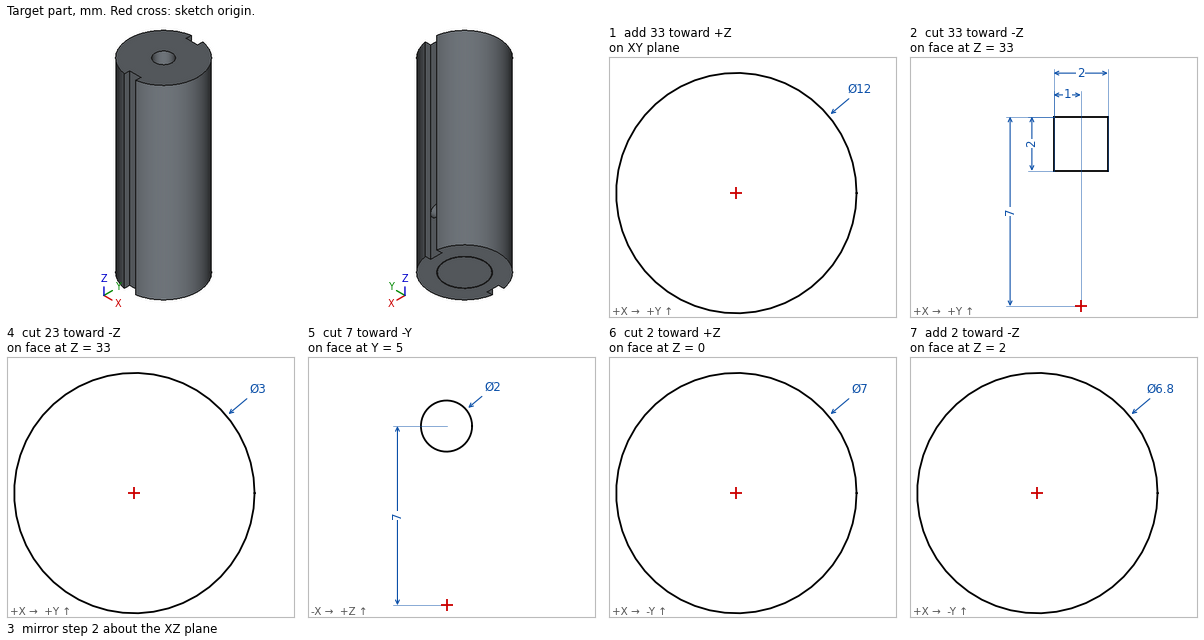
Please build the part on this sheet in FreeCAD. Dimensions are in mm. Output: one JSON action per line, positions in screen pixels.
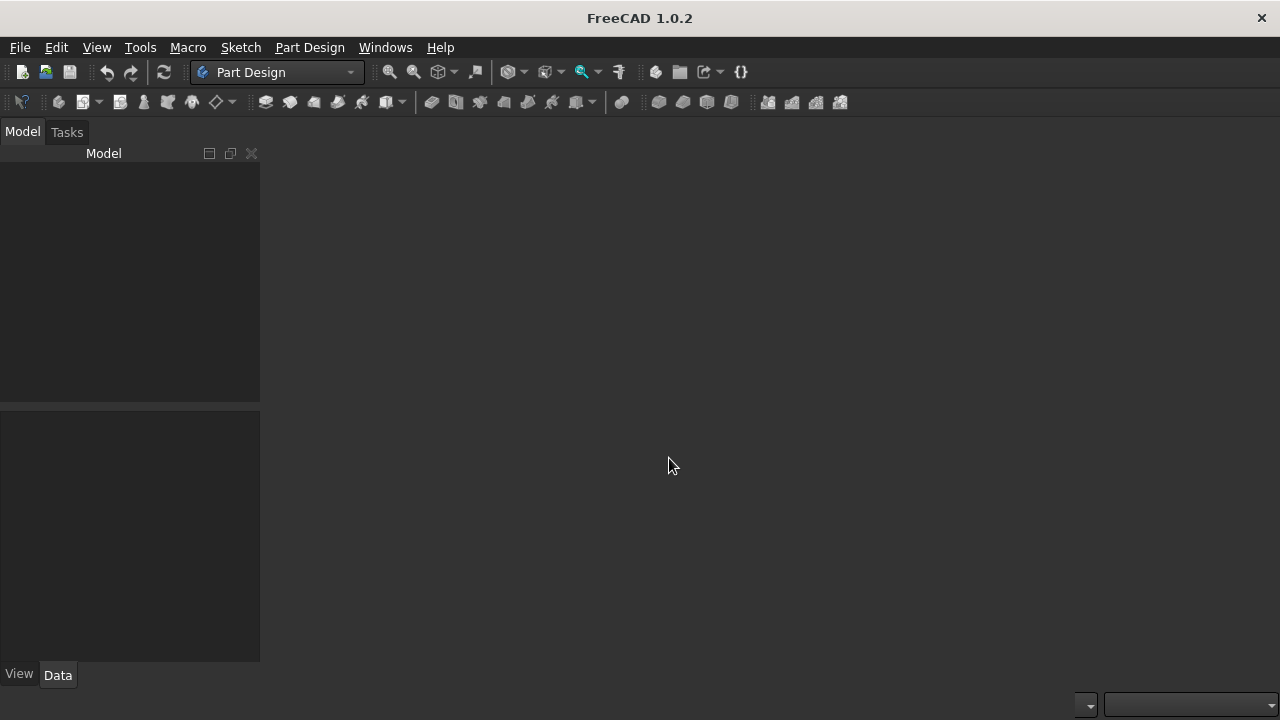
{"action": "key", "text": "ctrl+n"}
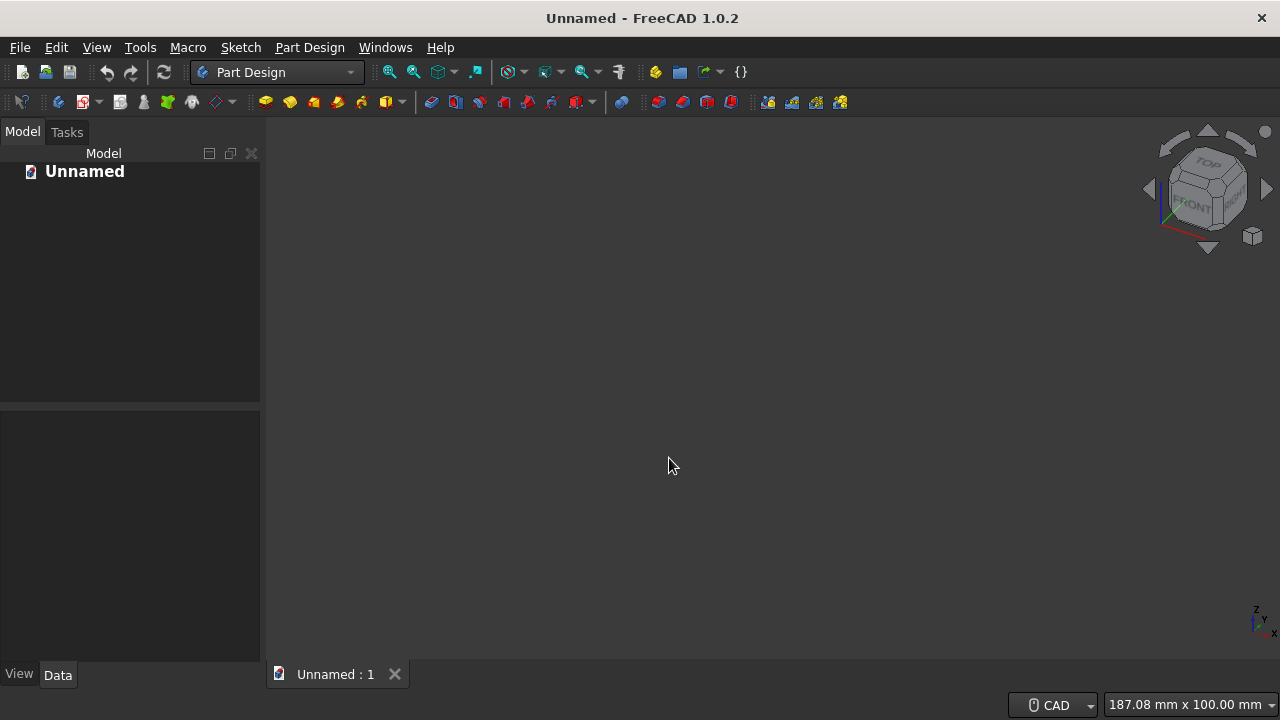
{"action": "left_click", "coordinate": [84, 102]}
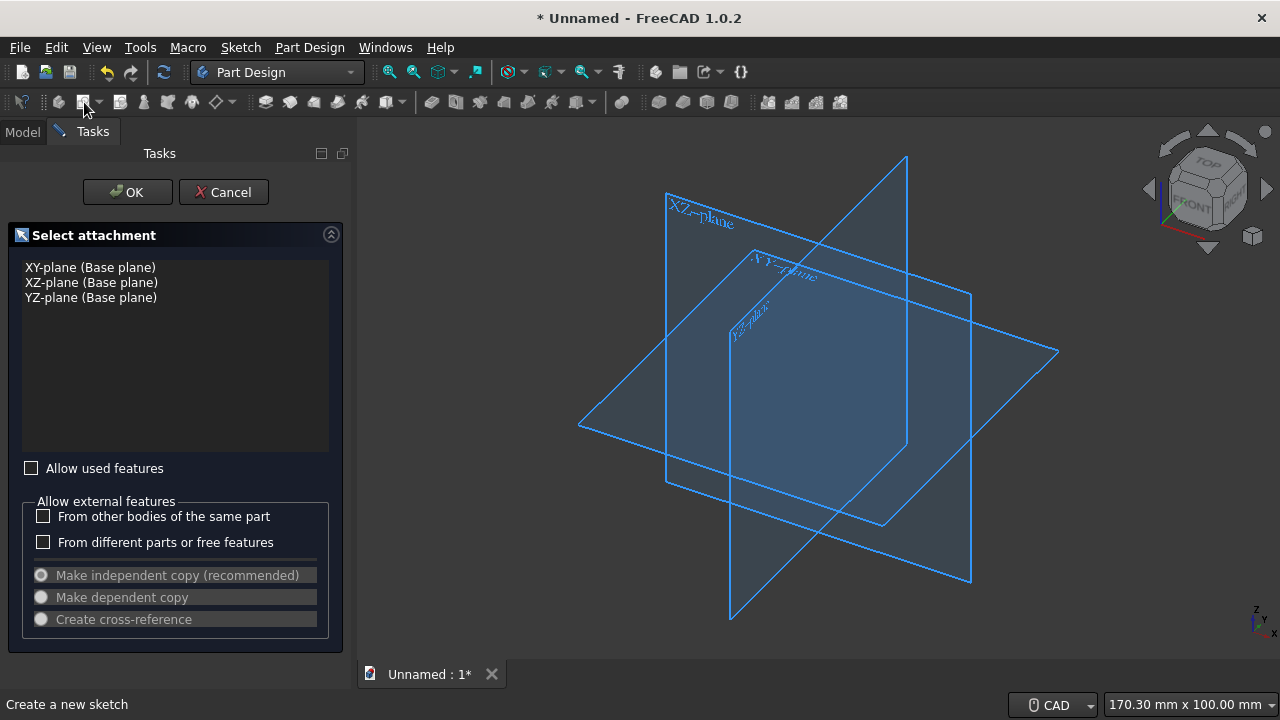
{"action": "left_click", "coordinate": [82, 268]}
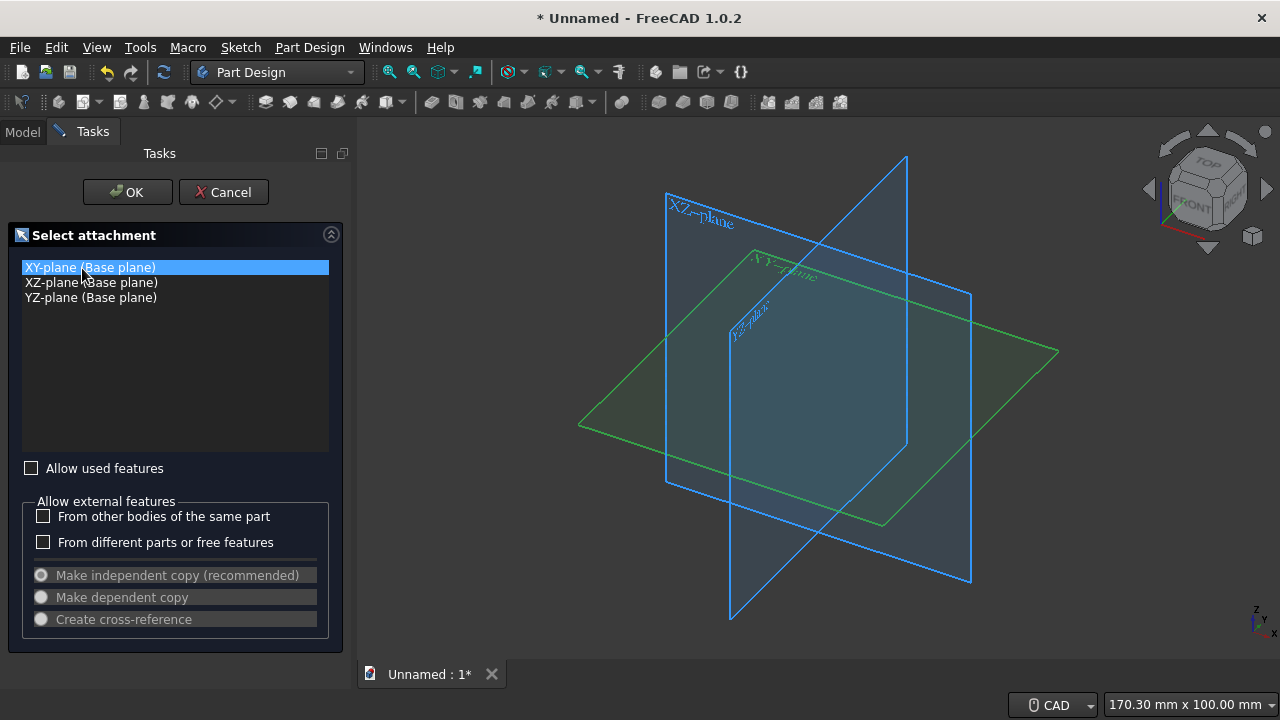
{"action": "left_click", "coordinate": [128, 192]}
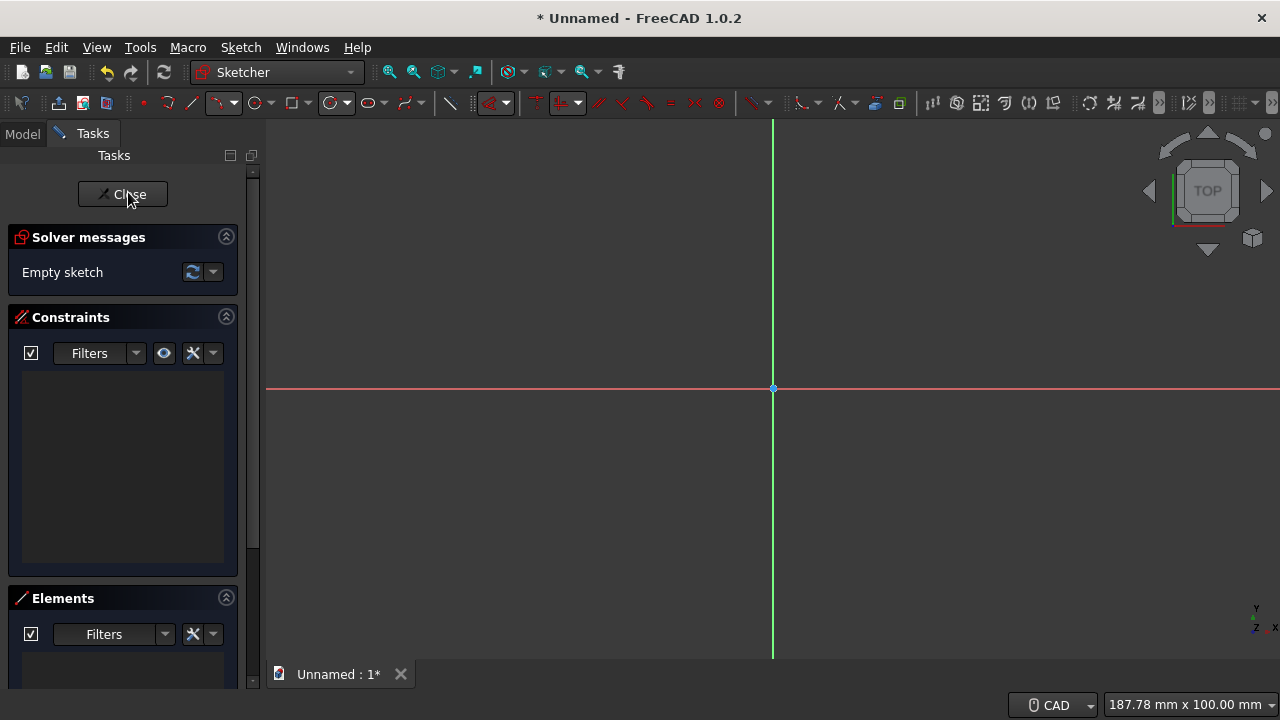
{"action": "scroll", "coordinate": [790, 389], "scroll_direction": "up", "scroll_amount": 8}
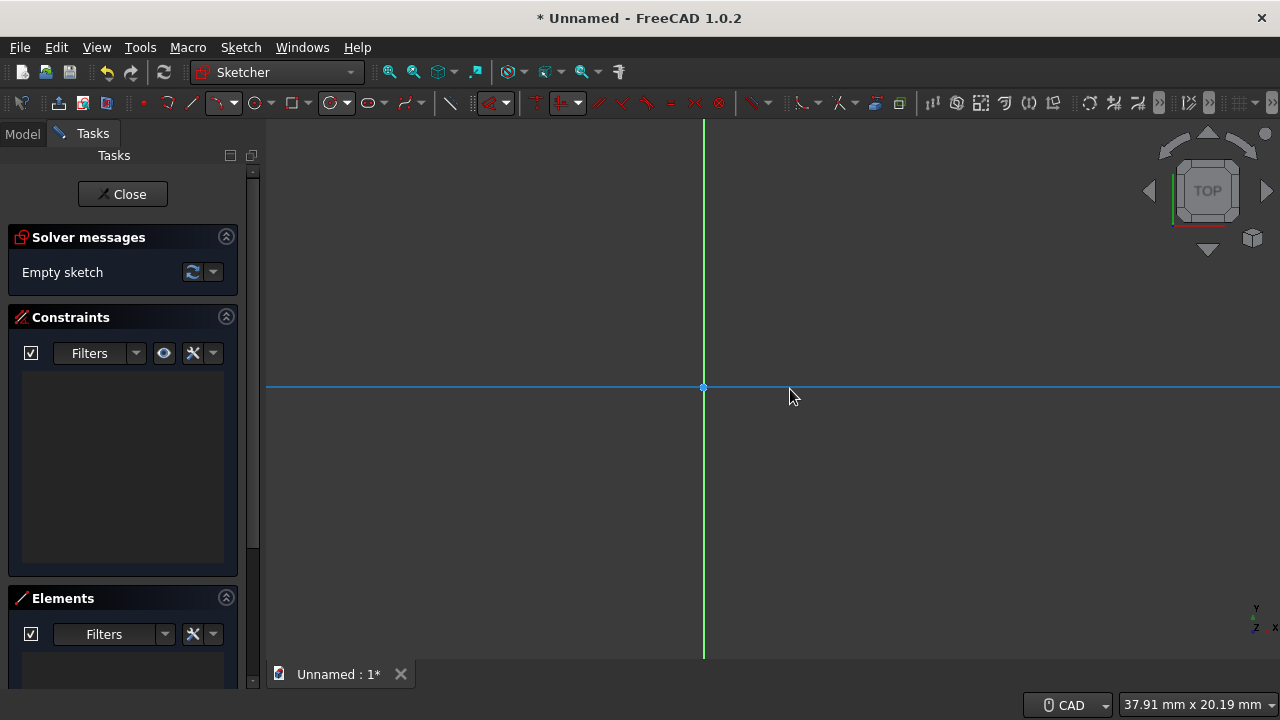
{"action": "key", "text": "g c"}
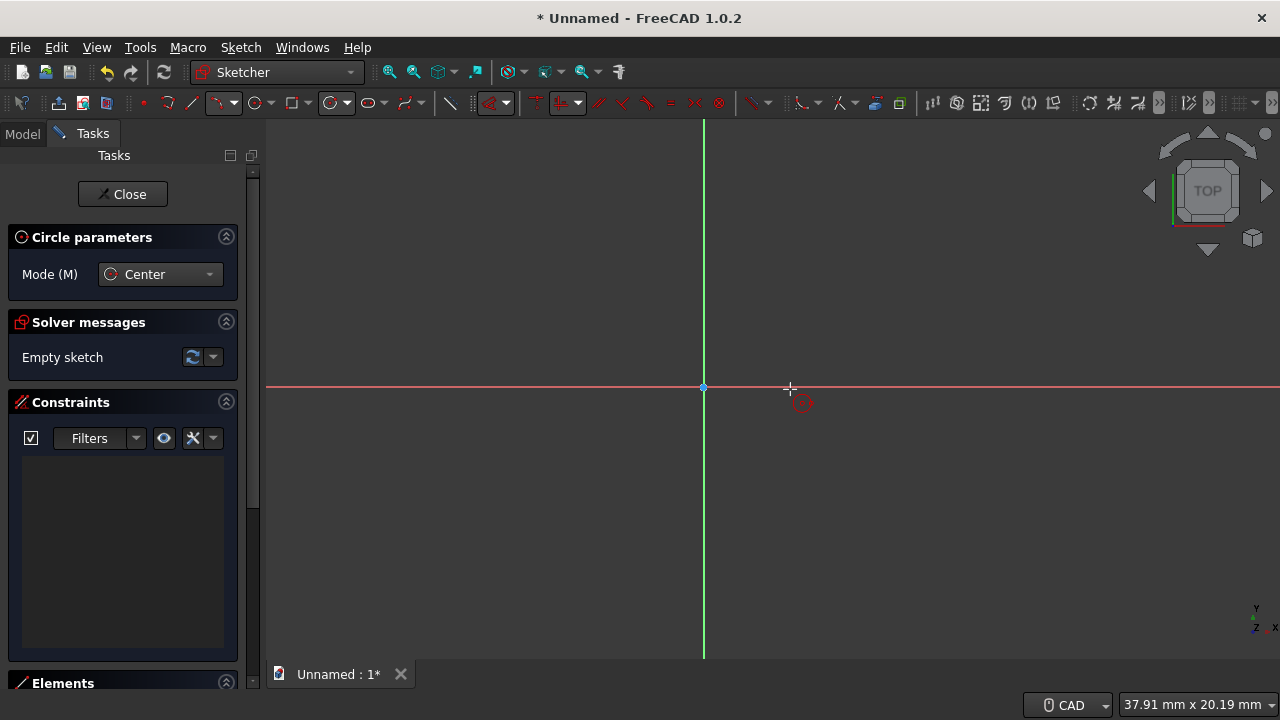
{"action": "left_click", "coordinate": [704, 387]}
{"action": "left_click", "coordinate": [817, 274]}
{"action": "key", "text": "Escape"}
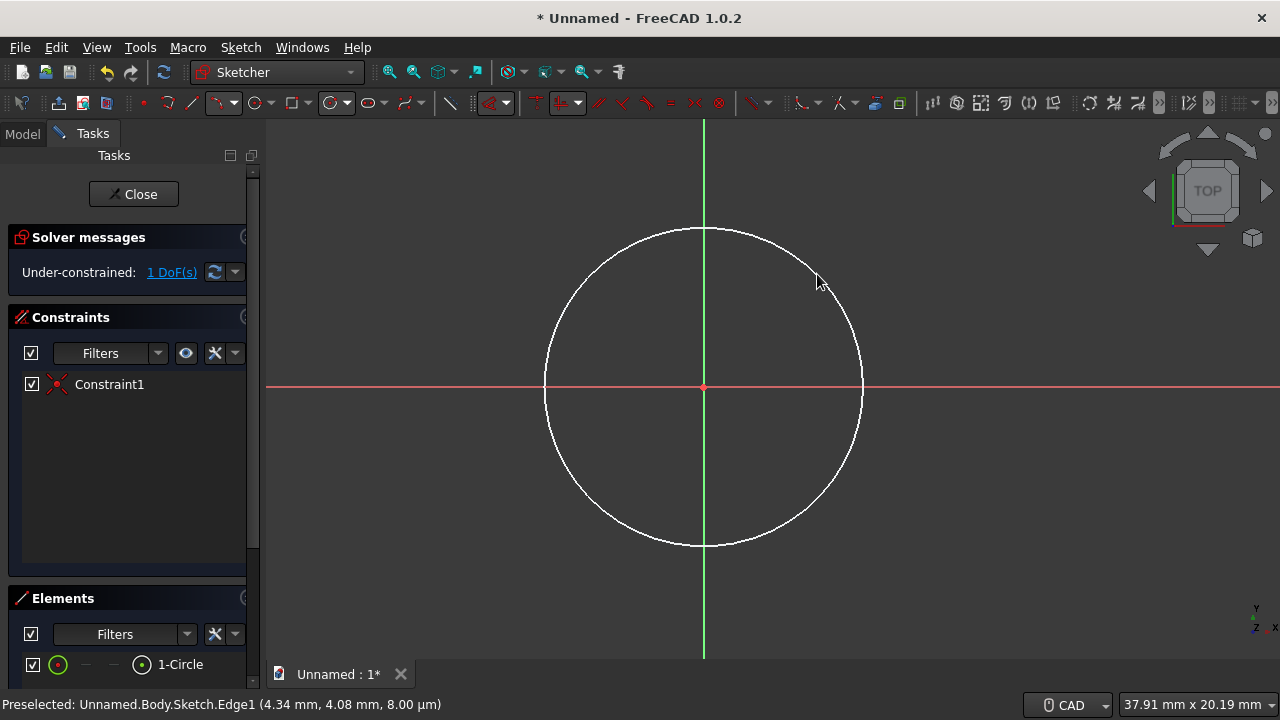
{"action": "key", "text": "d"}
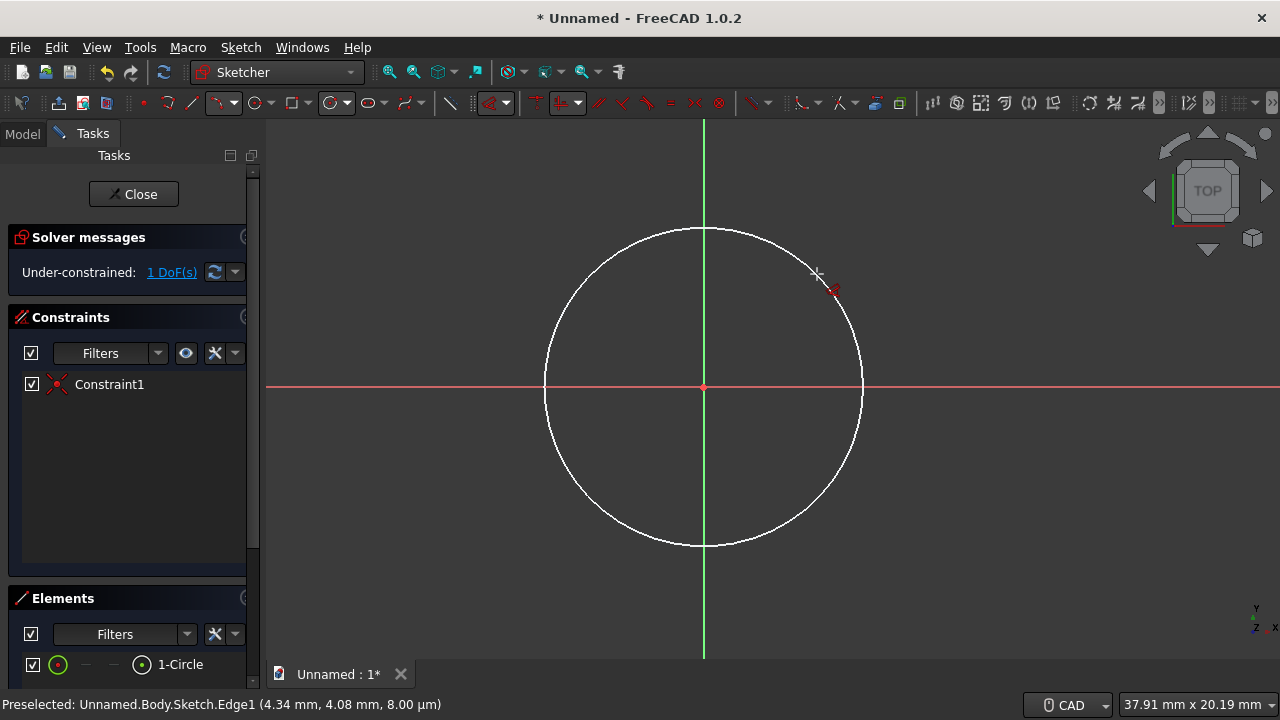
{"action": "left_click", "coordinate": [816, 274]}
{"action": "left_click", "coordinate": [839, 251]}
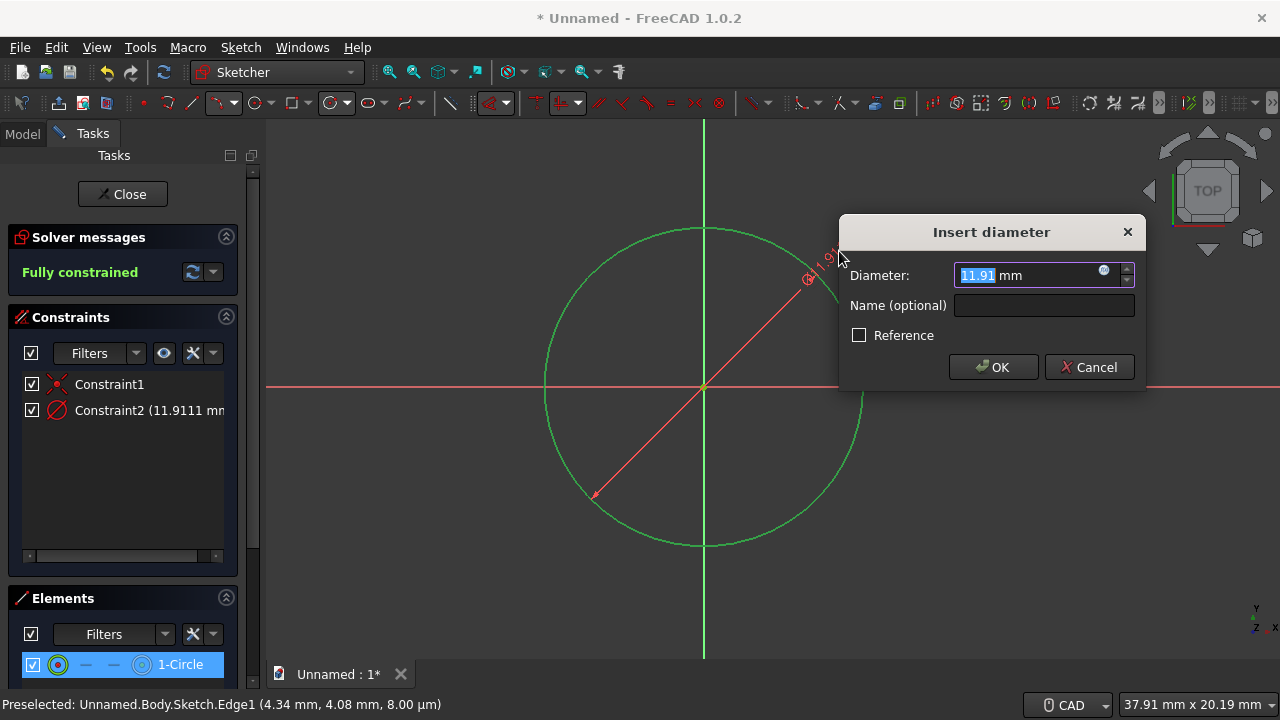
{"action": "type", "text": "12"}
{"action": "key", "text": "Return"}
{"action": "key", "text": "Escape"}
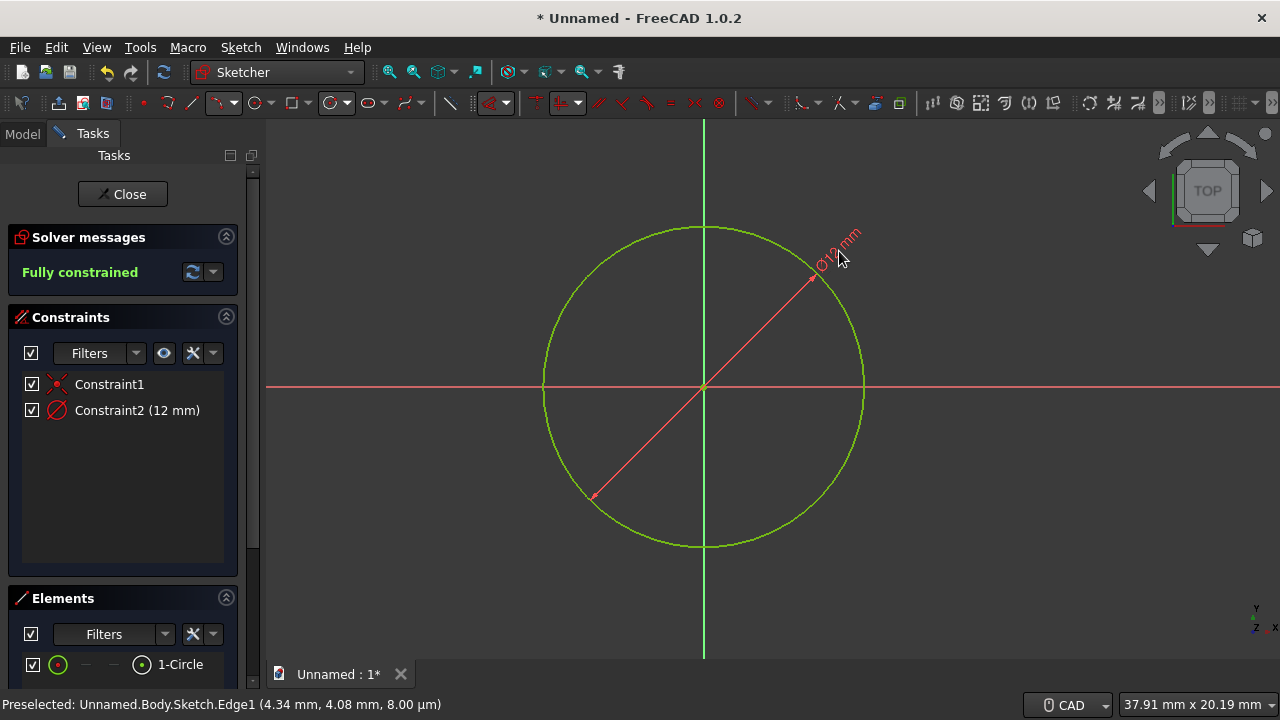
{"action": "left_click", "coordinate": [123, 194]}